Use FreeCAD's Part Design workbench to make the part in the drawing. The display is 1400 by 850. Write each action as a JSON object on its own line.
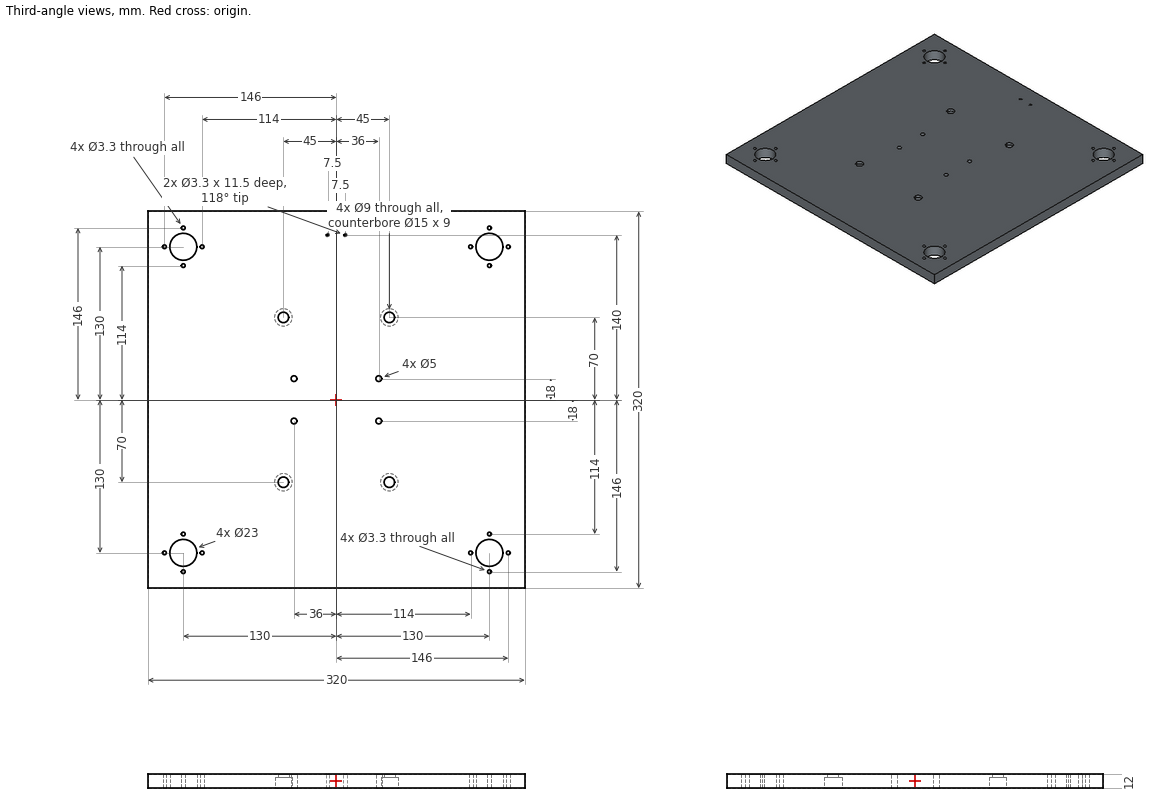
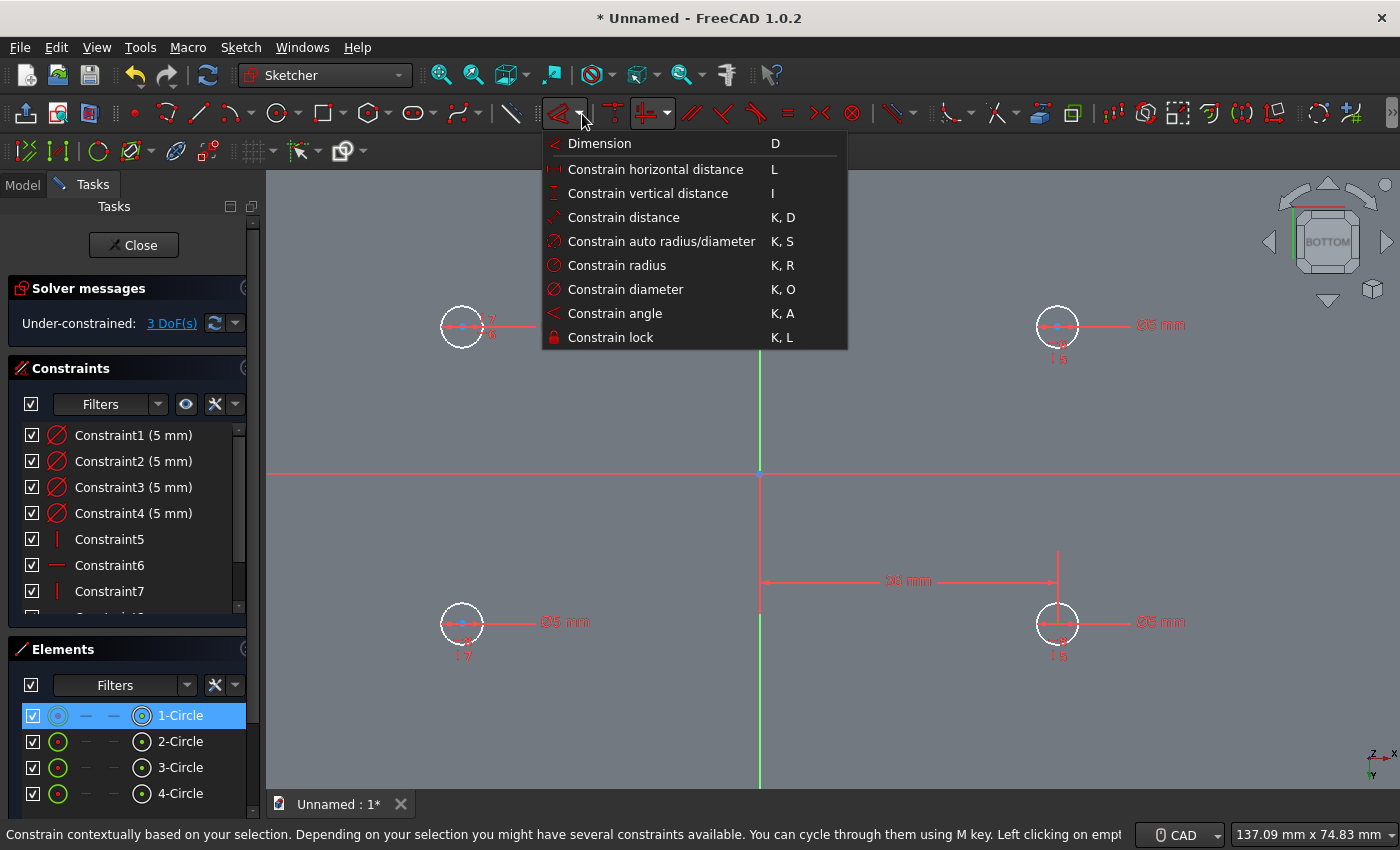
{"action": "left_click", "coordinate": [695, 193]}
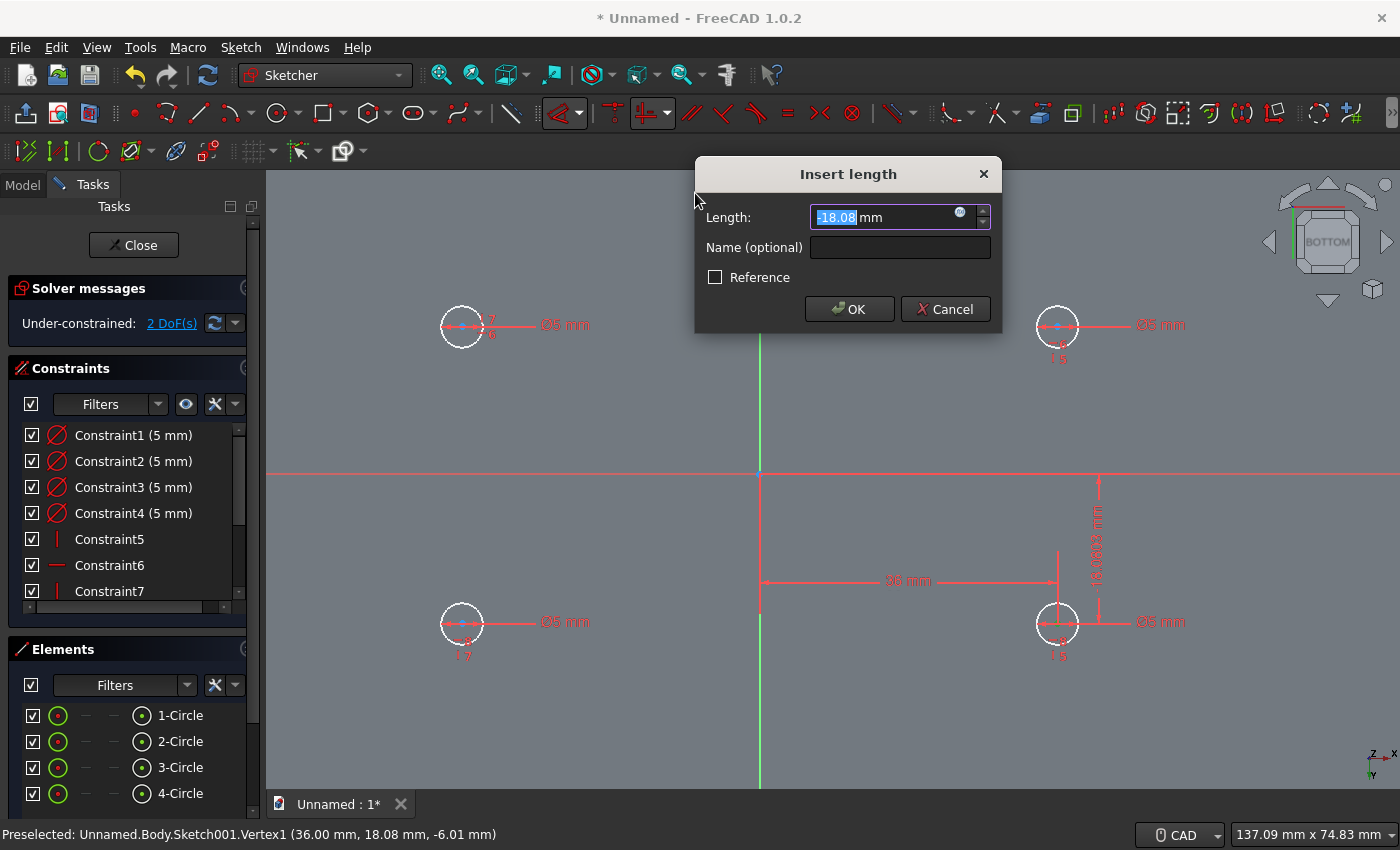
{"action": "type", "text": "-18"}
{"action": "key", "text": "Return"}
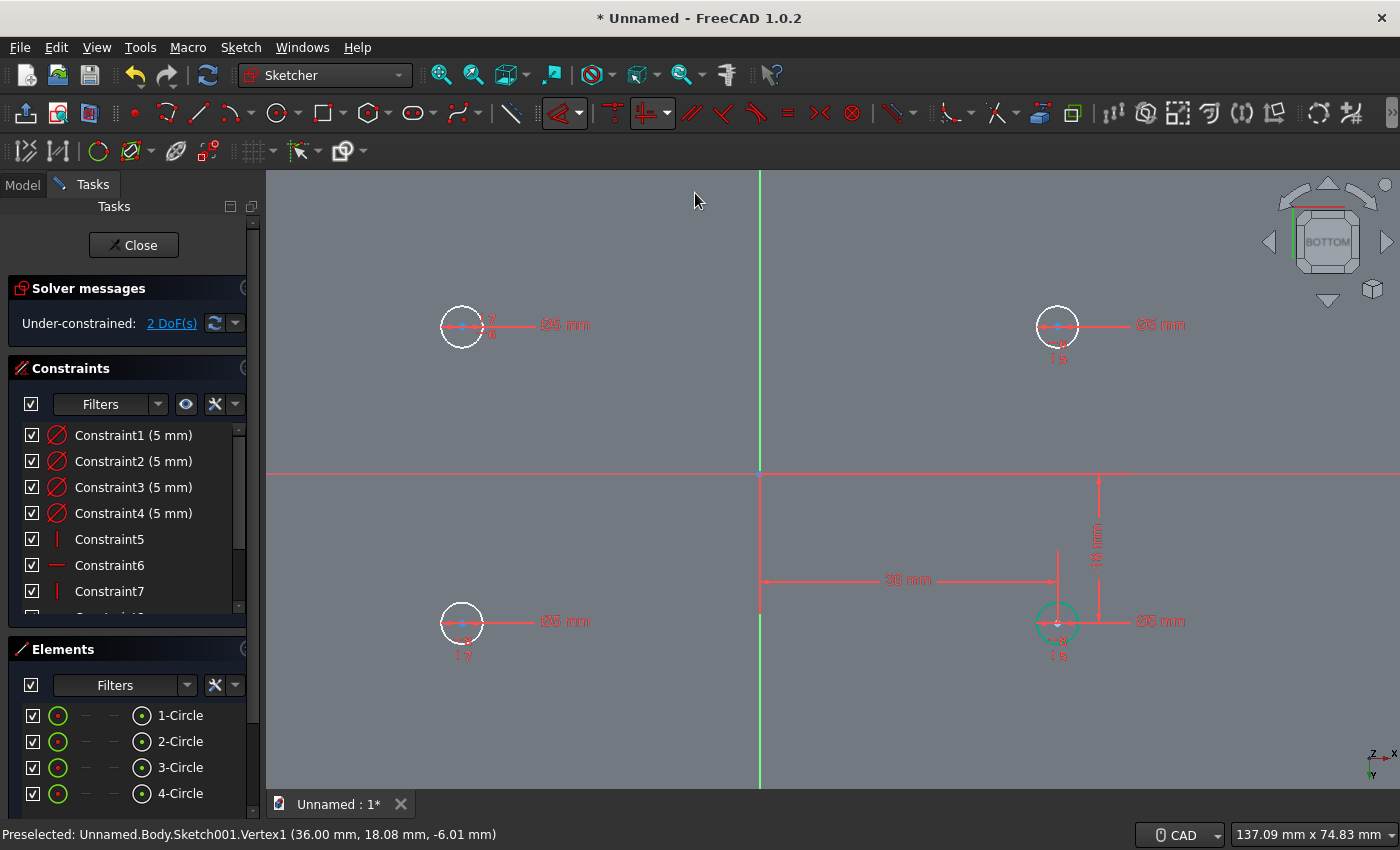
{"action": "left_click", "coordinate": [1058, 327]}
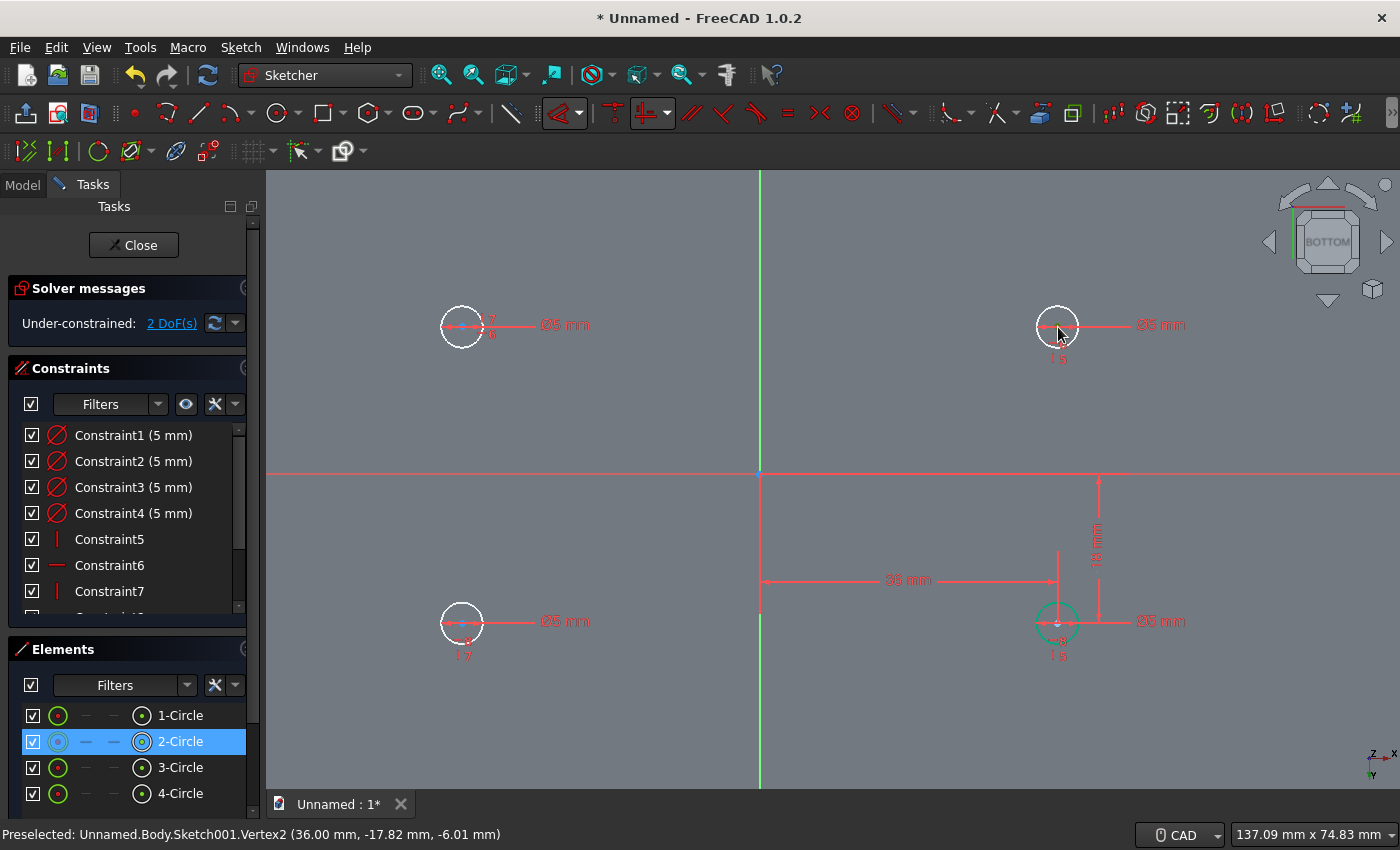
{"action": "key", "text": "i"}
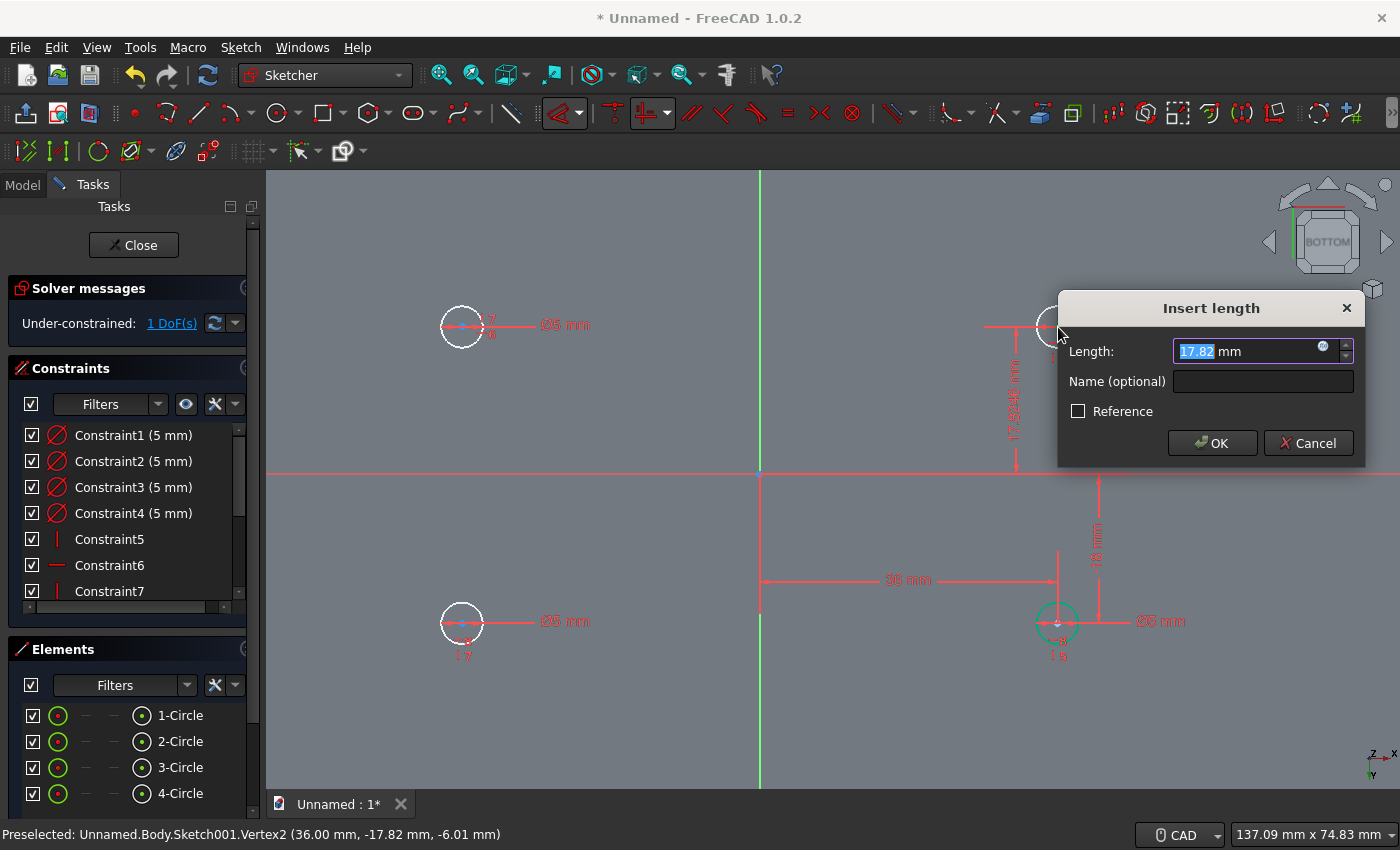
{"action": "type", "text": "18"}
{"action": "key", "text": "Return"}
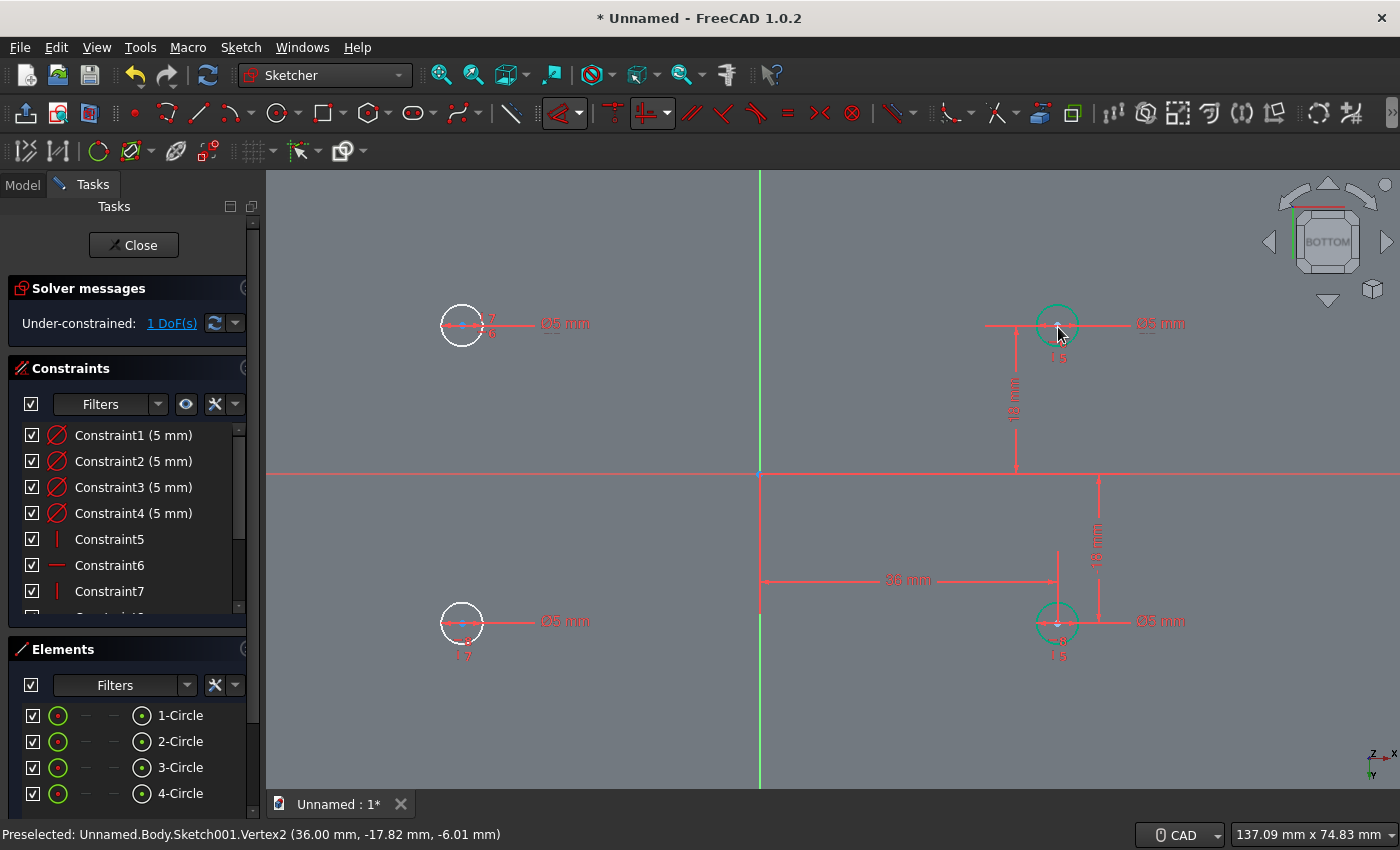
{"action": "left_click", "coordinate": [462, 326]}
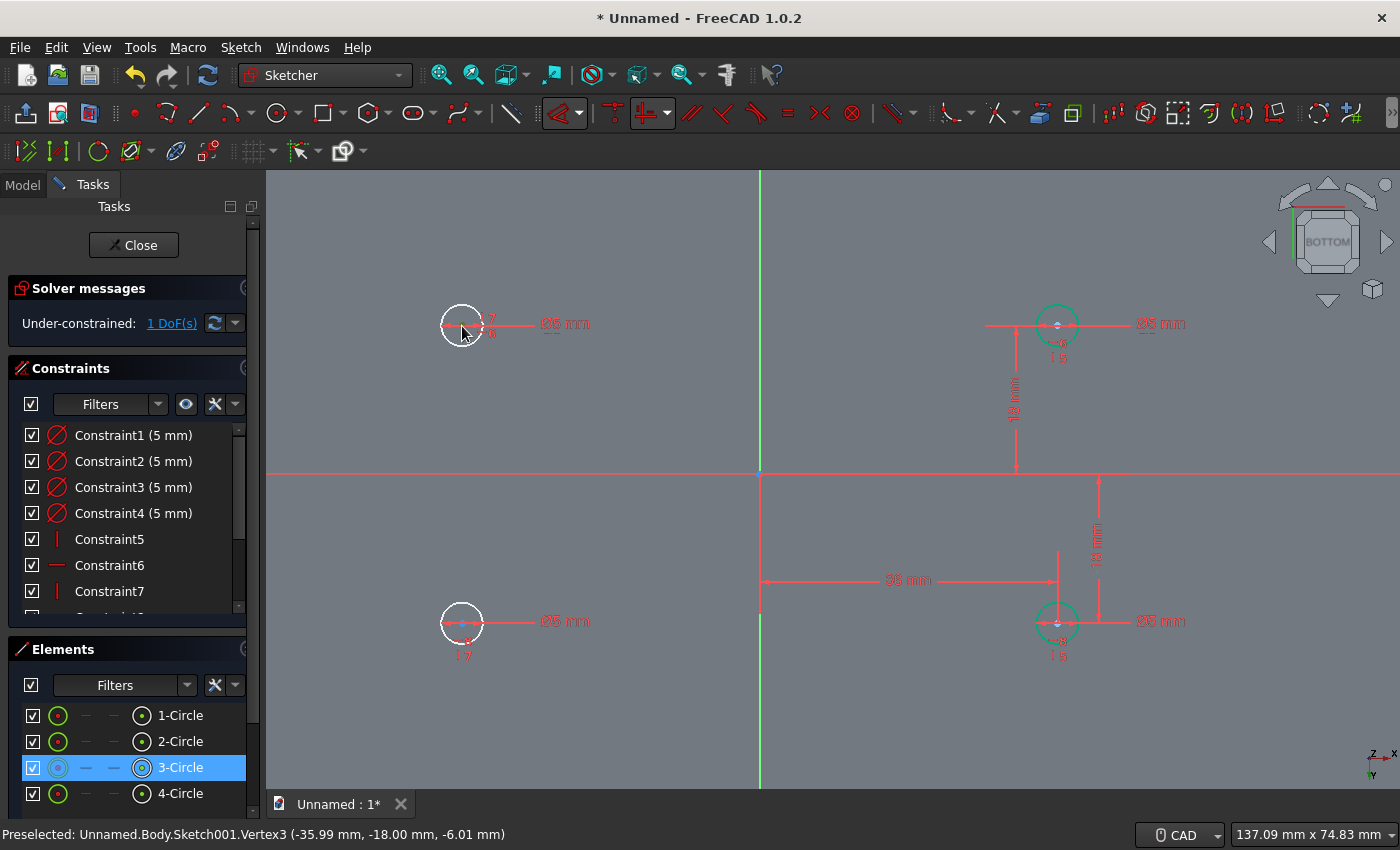
{"action": "left_click", "coordinate": [582, 114]}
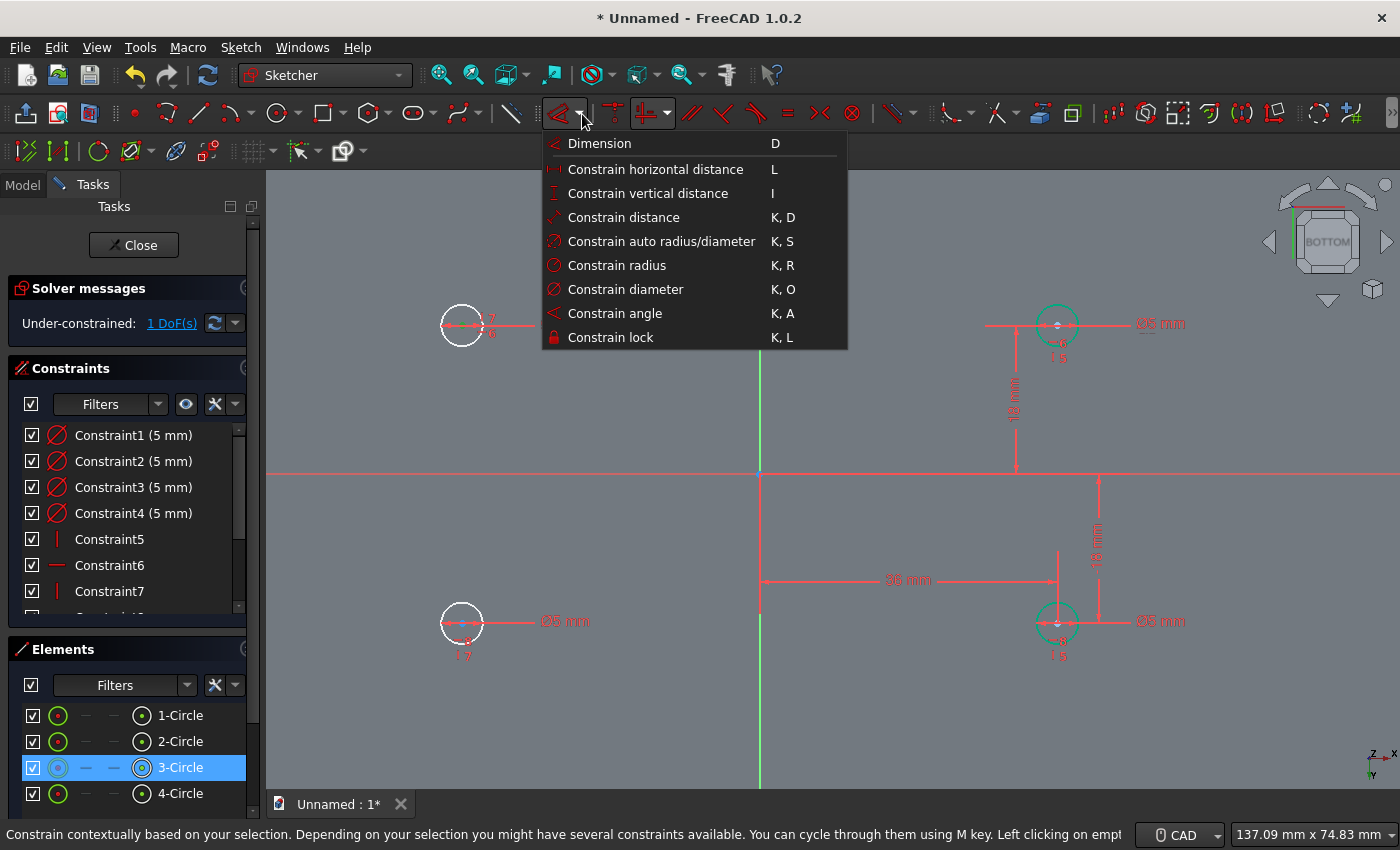
{"action": "left_click", "coordinate": [695, 169]}